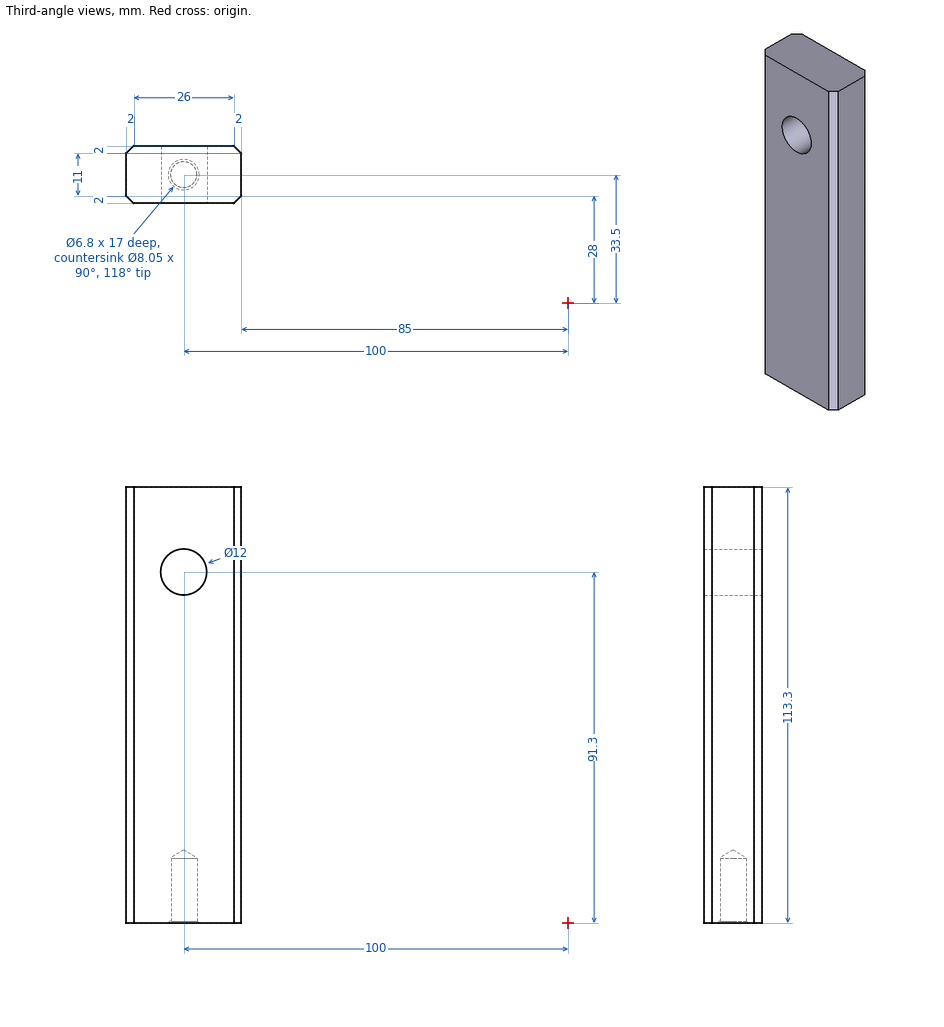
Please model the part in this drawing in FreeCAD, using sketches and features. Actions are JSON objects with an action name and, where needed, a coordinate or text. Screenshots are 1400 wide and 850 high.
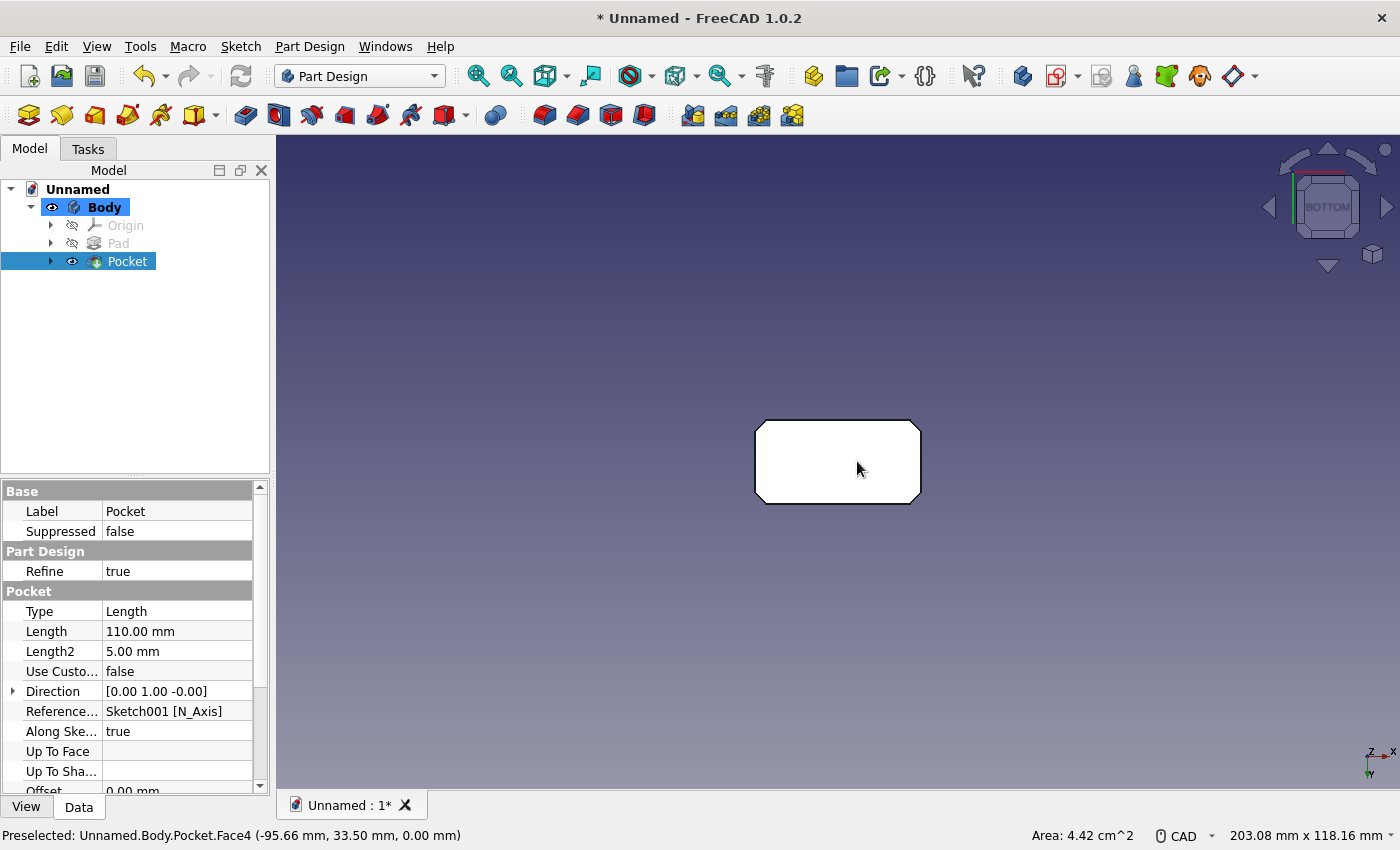
{"action": "left_click", "coordinate": [1056, 76]}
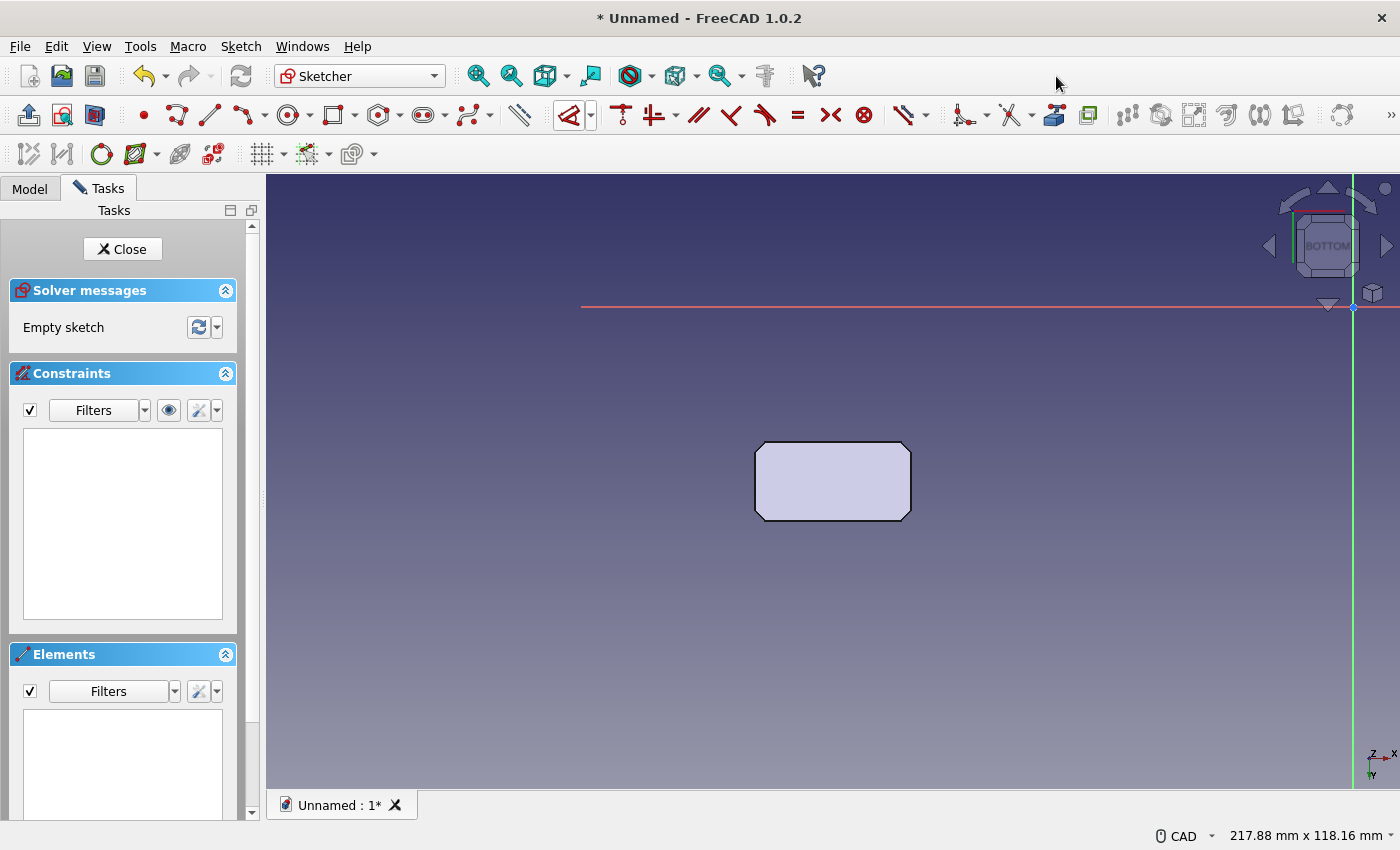
{"action": "scroll", "coordinate": [840, 481], "scroll_direction": "up", "scroll_amount": 12}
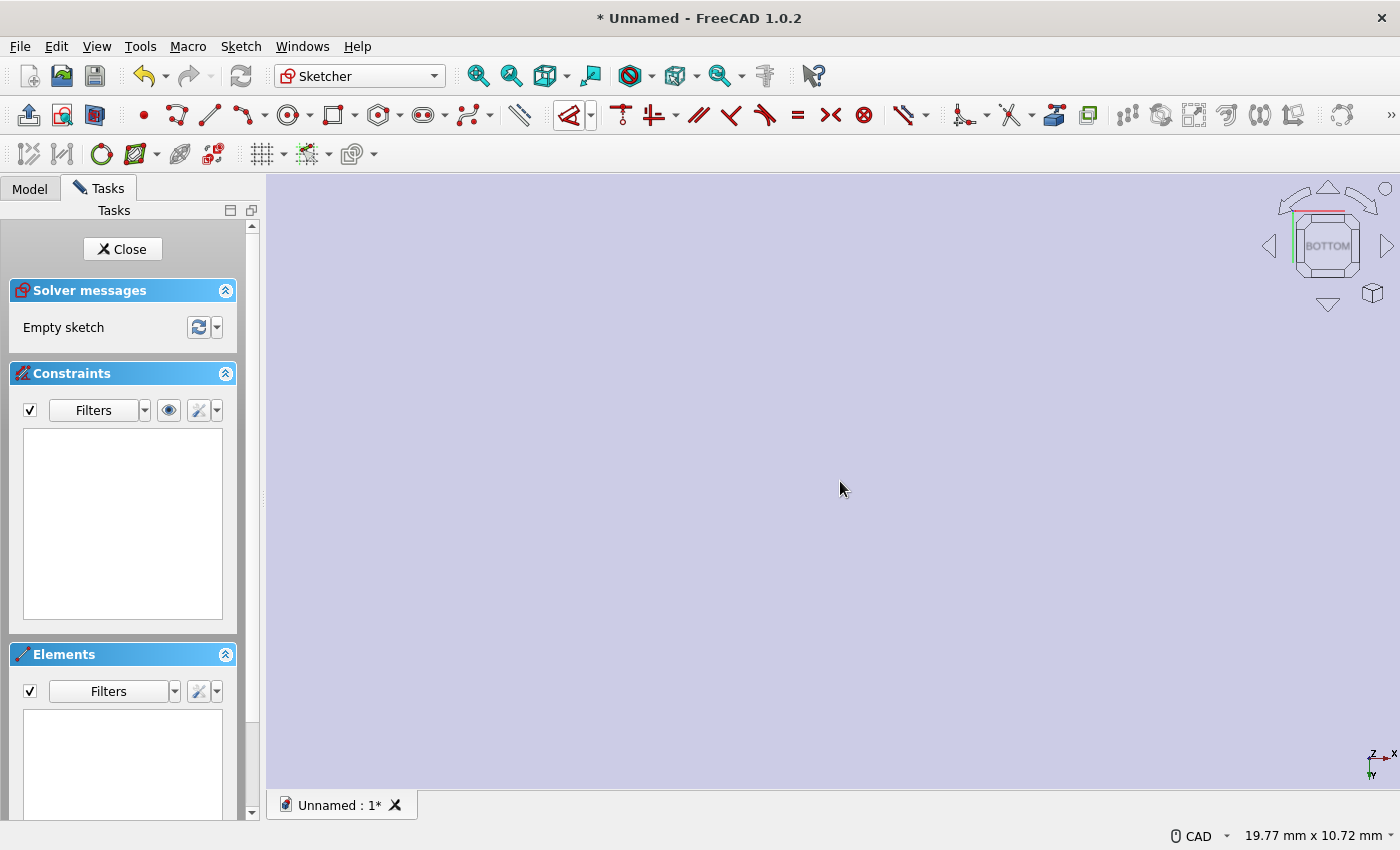
{"action": "left_click", "coordinate": [288, 116]}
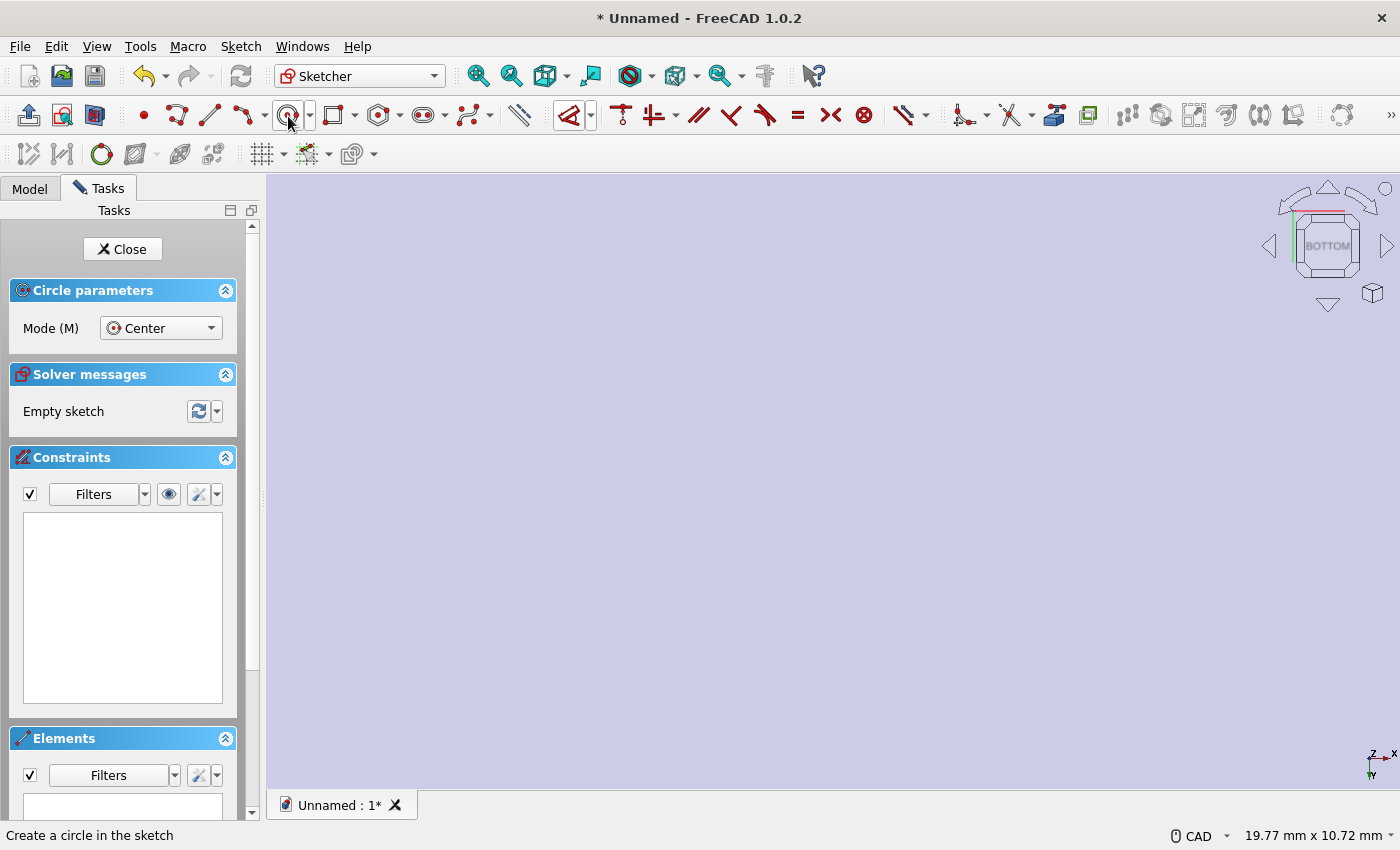
{"action": "left_click", "coordinate": [758, 482]}
{"action": "left_click", "coordinate": [896, 344]}
{"action": "key", "text": "Escape"}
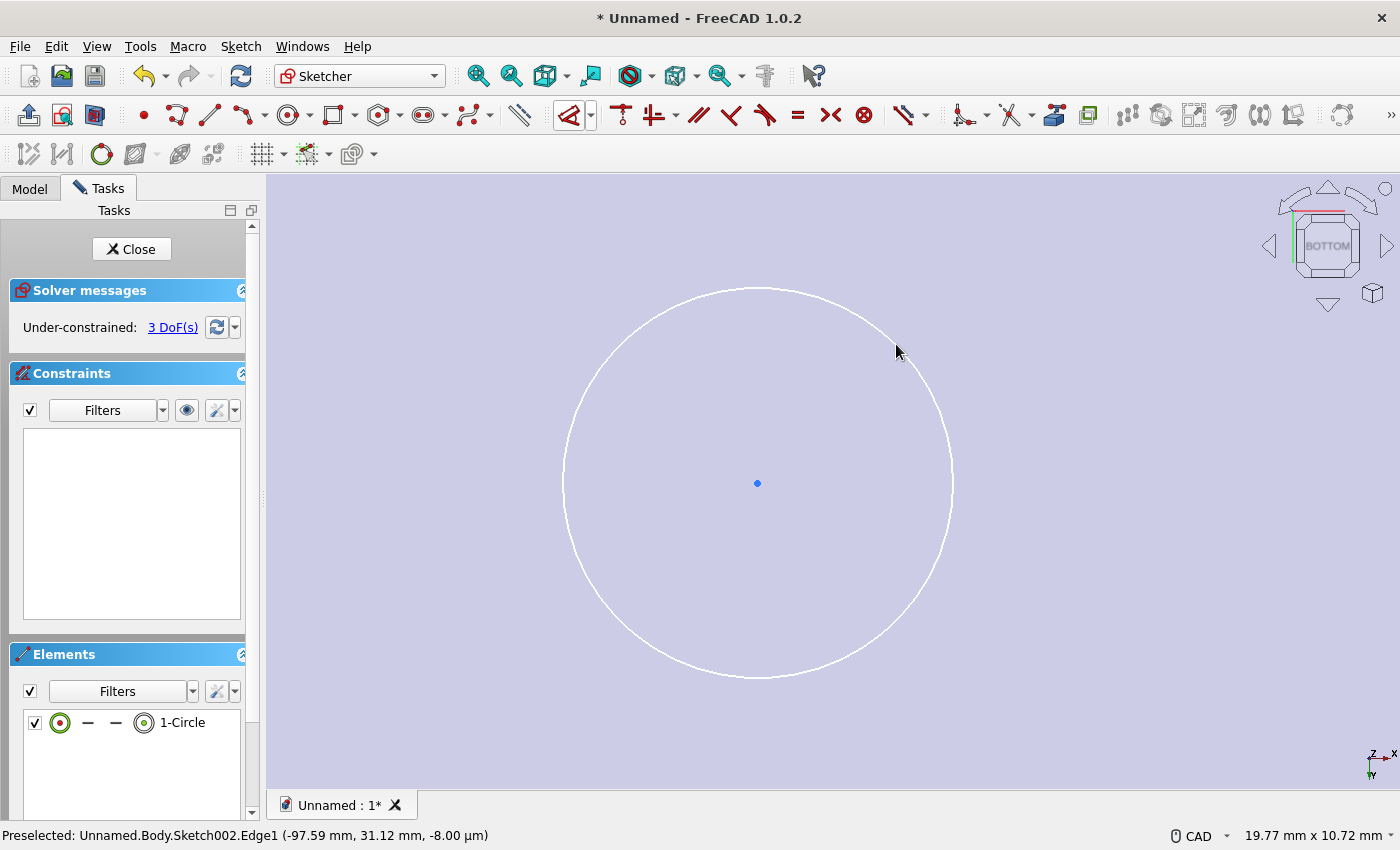
{"action": "left_click", "coordinate": [896, 345]}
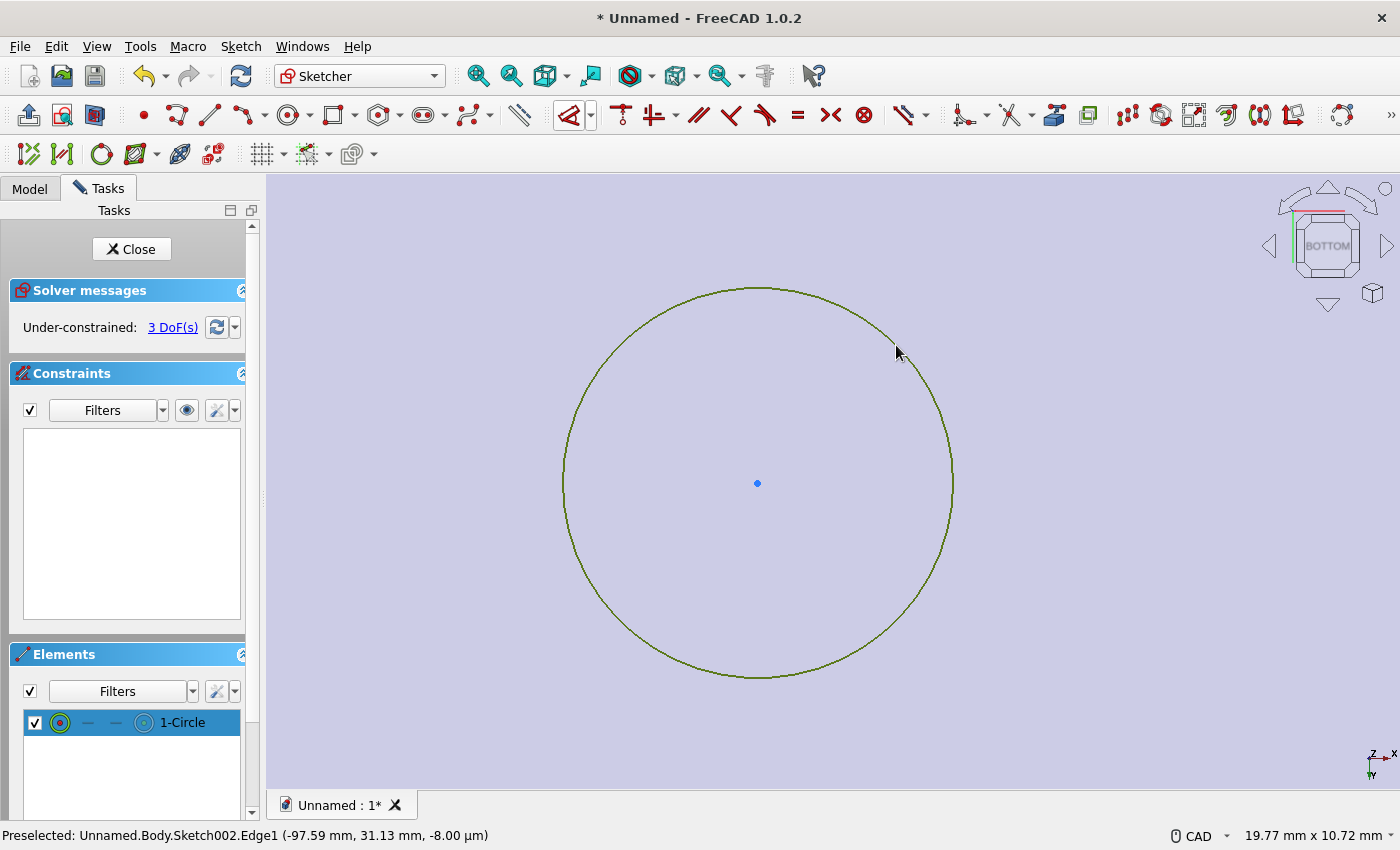
{"action": "left_click", "coordinate": [590, 116]}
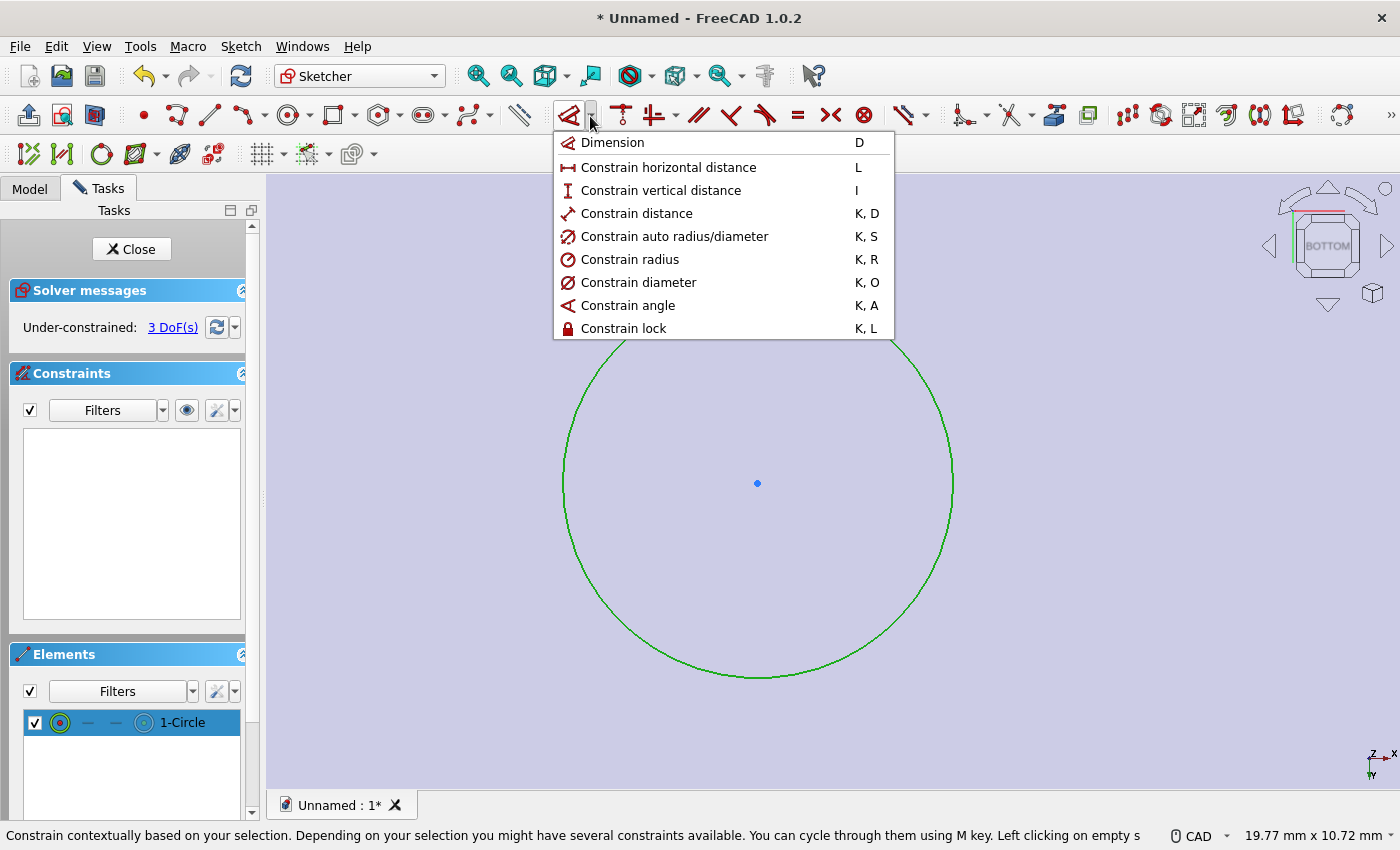
{"action": "left_click", "coordinate": [724, 282]}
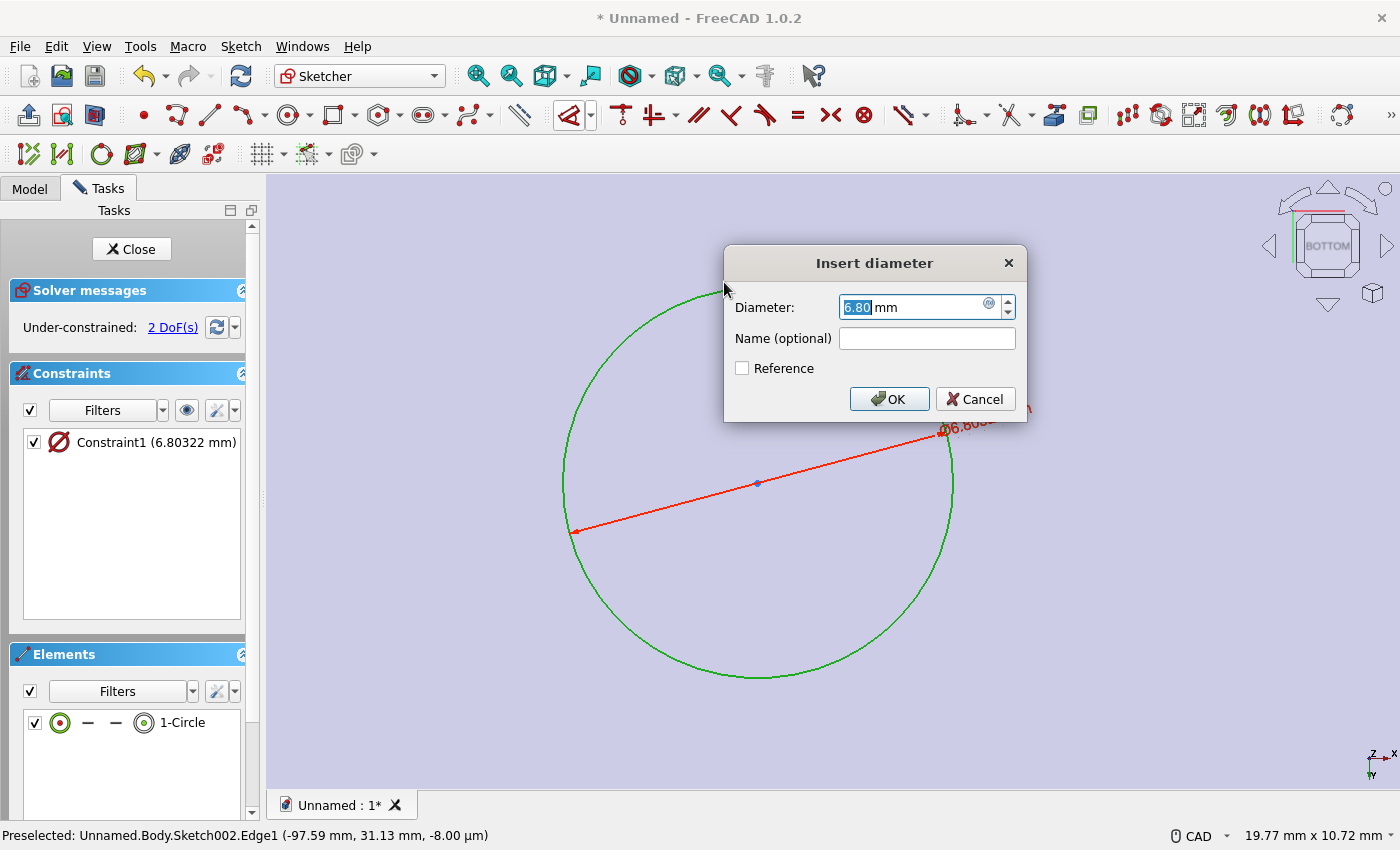
{"action": "type", "text": "6.8"}
{"action": "key", "text": "Return"}